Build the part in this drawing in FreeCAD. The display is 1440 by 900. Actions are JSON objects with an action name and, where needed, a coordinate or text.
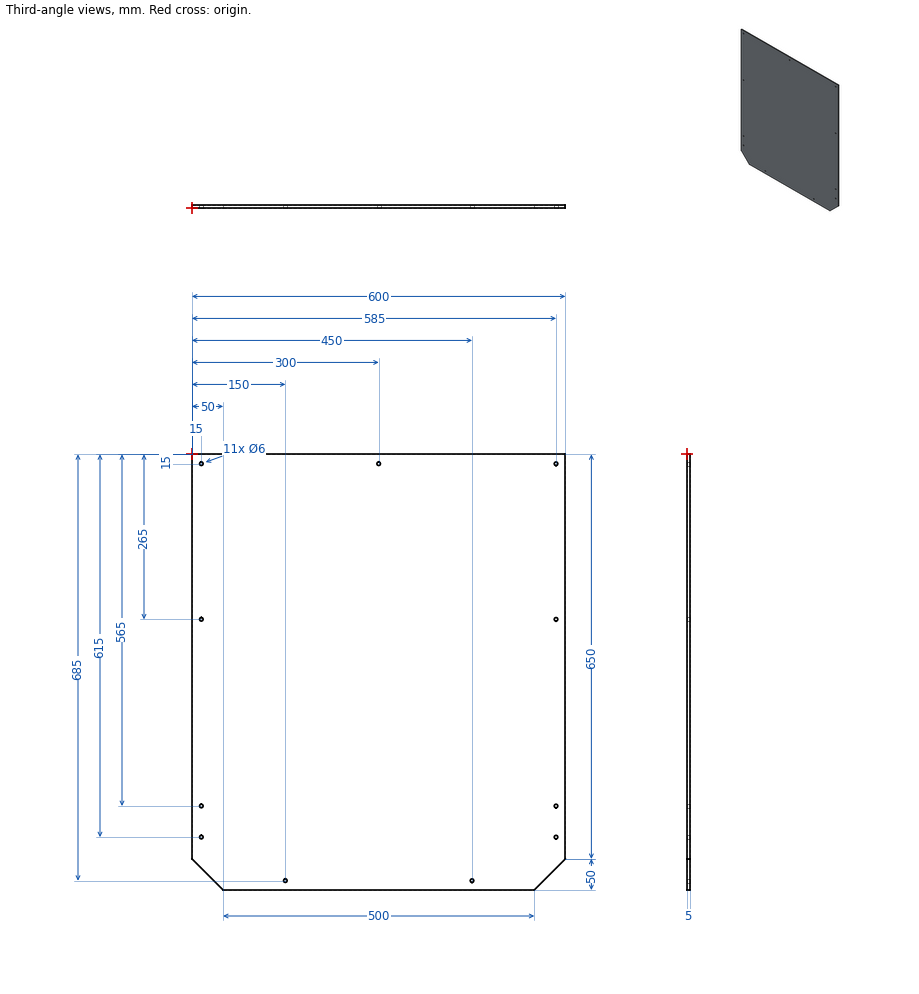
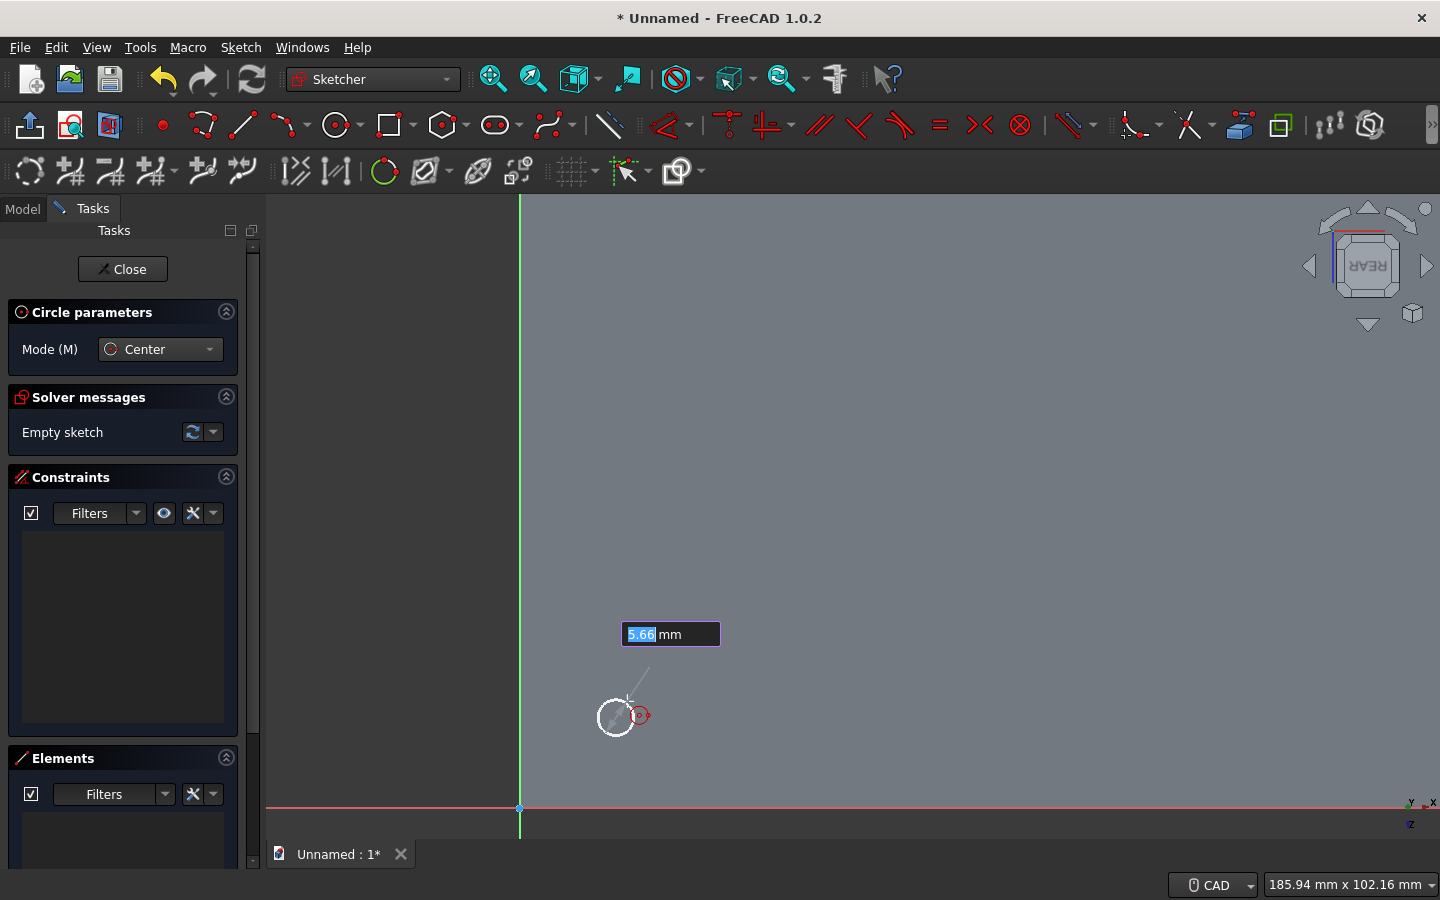
{"action": "left_click", "coordinate": [628, 700]}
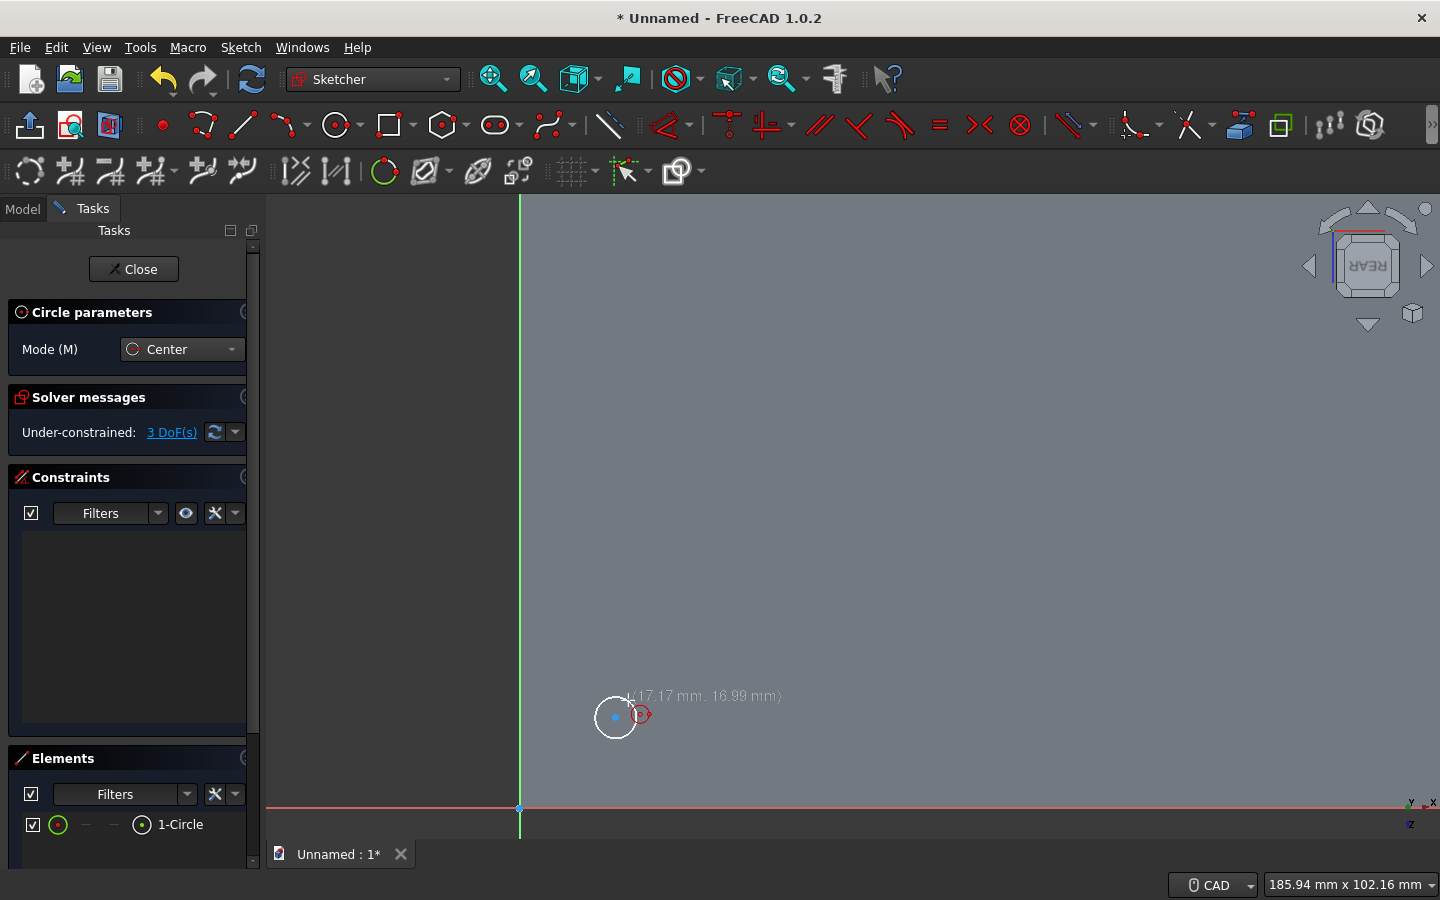
{"action": "scroll", "coordinate": [626, 704], "scroll_direction": "down", "scroll_amount": 12}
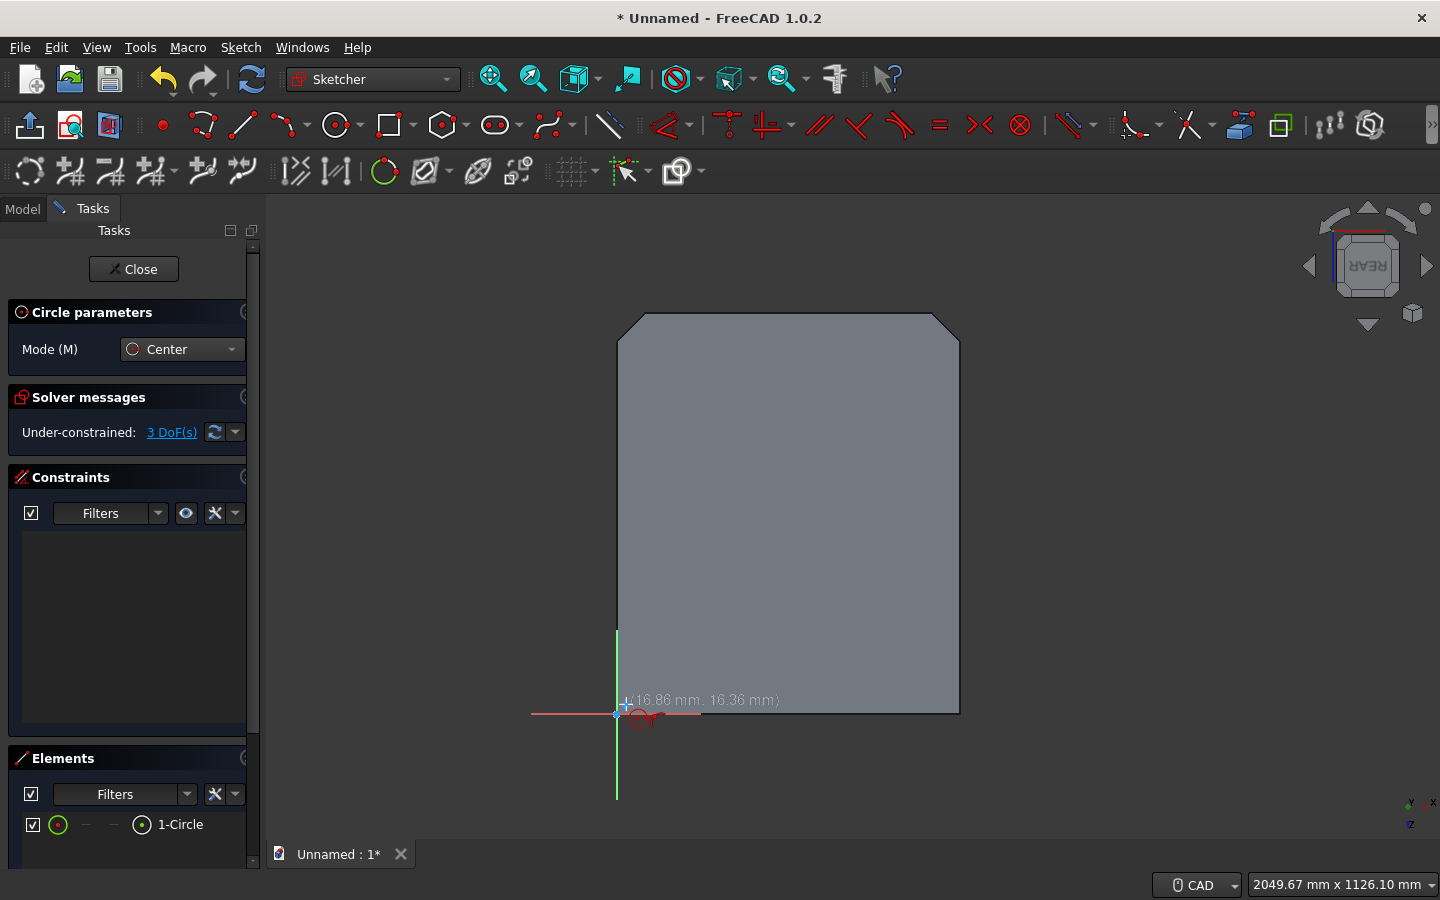
{"action": "scroll", "coordinate": [625, 562], "scroll_direction": "up", "scroll_amount": 13}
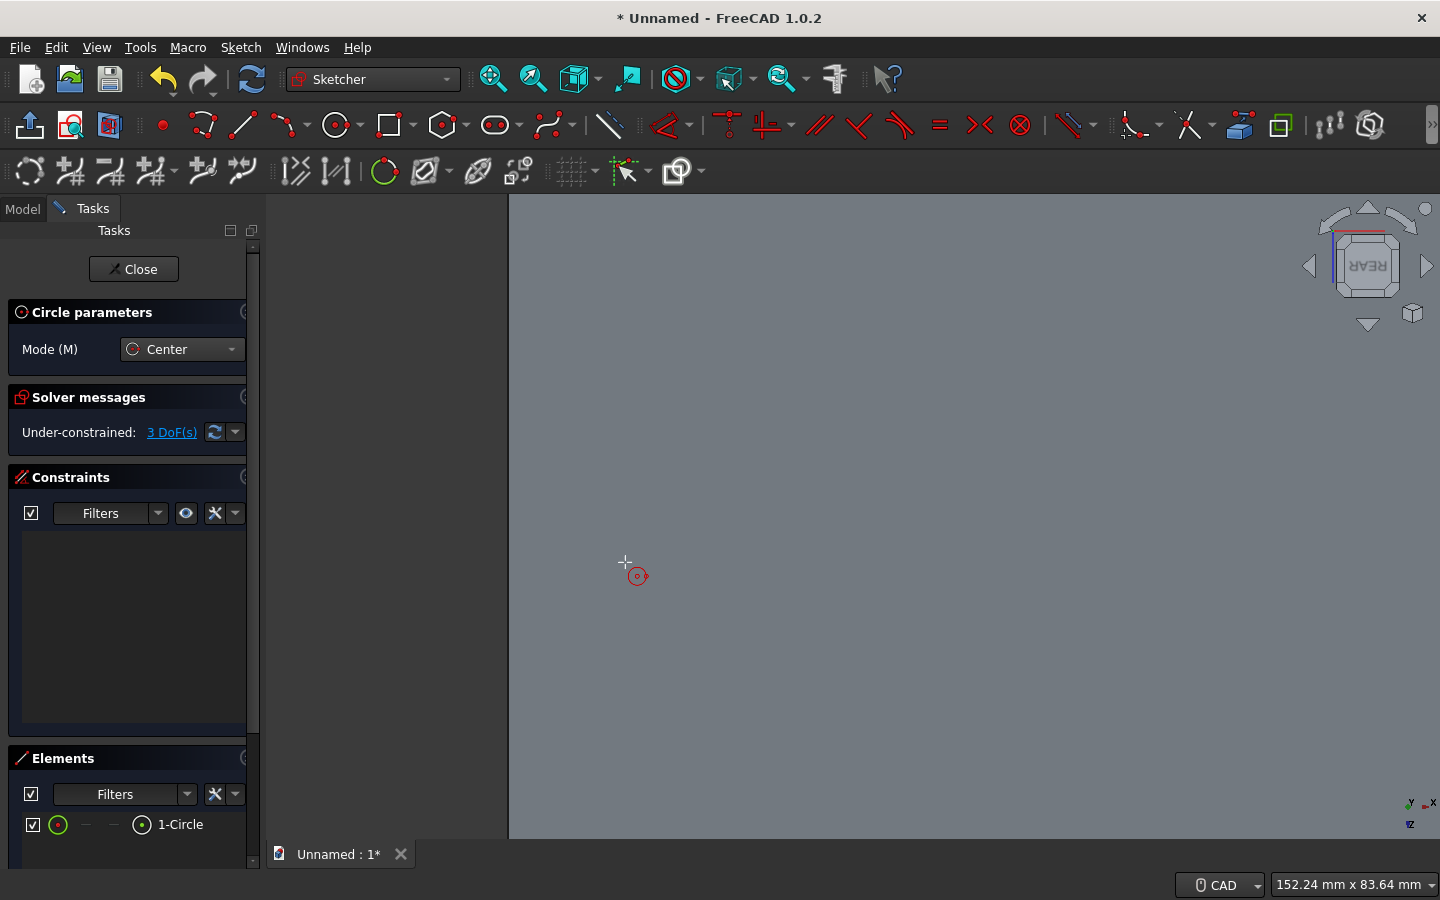
{"action": "scroll", "coordinate": [625, 562], "scroll_direction": "down", "scroll_amount": 13}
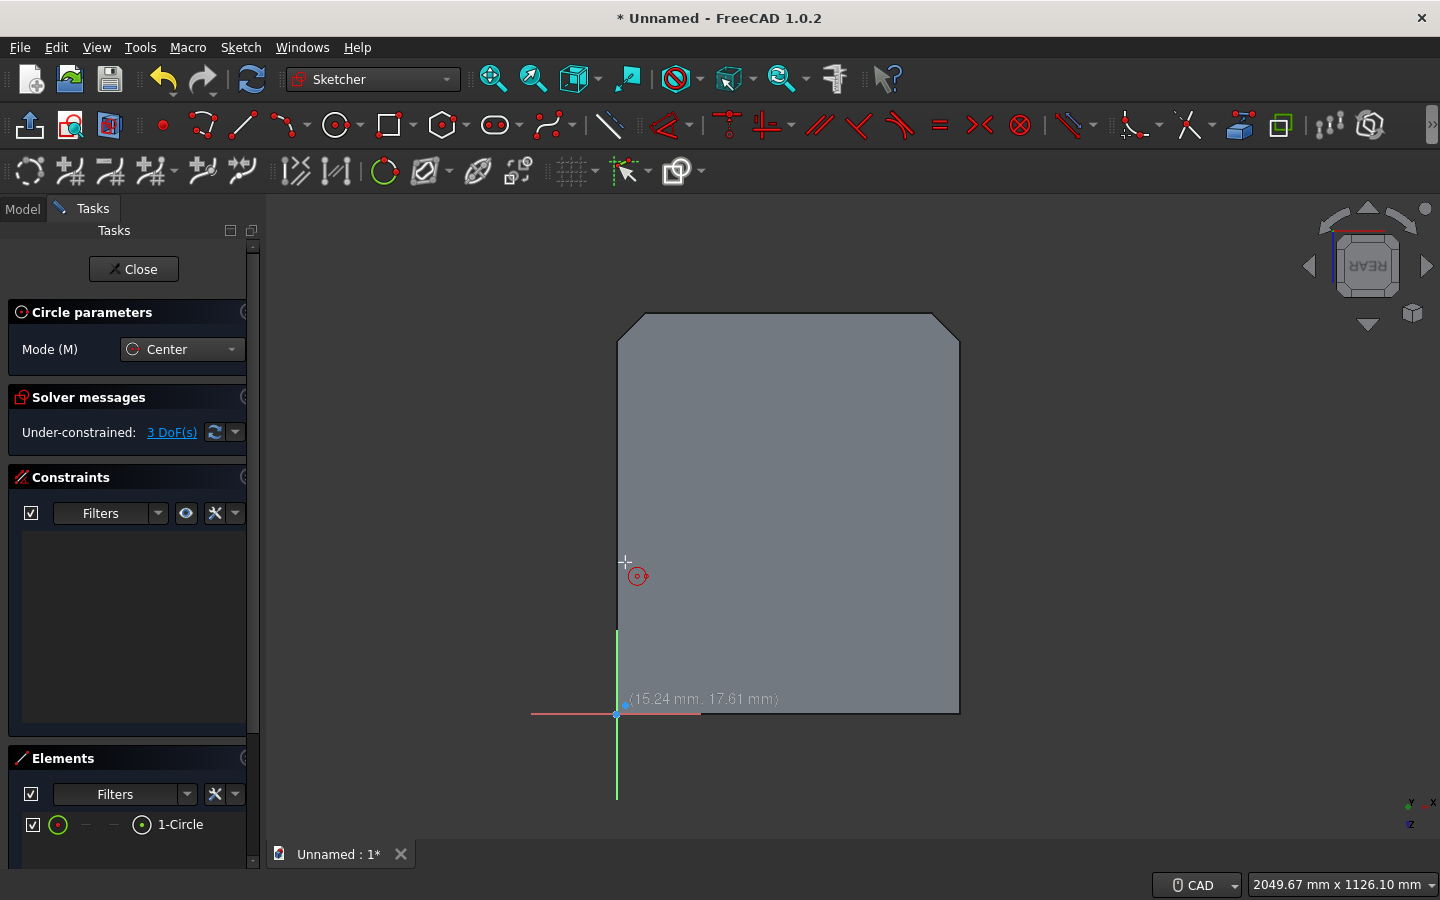
{"action": "scroll", "coordinate": [625, 562], "scroll_direction": "up", "scroll_amount": 4}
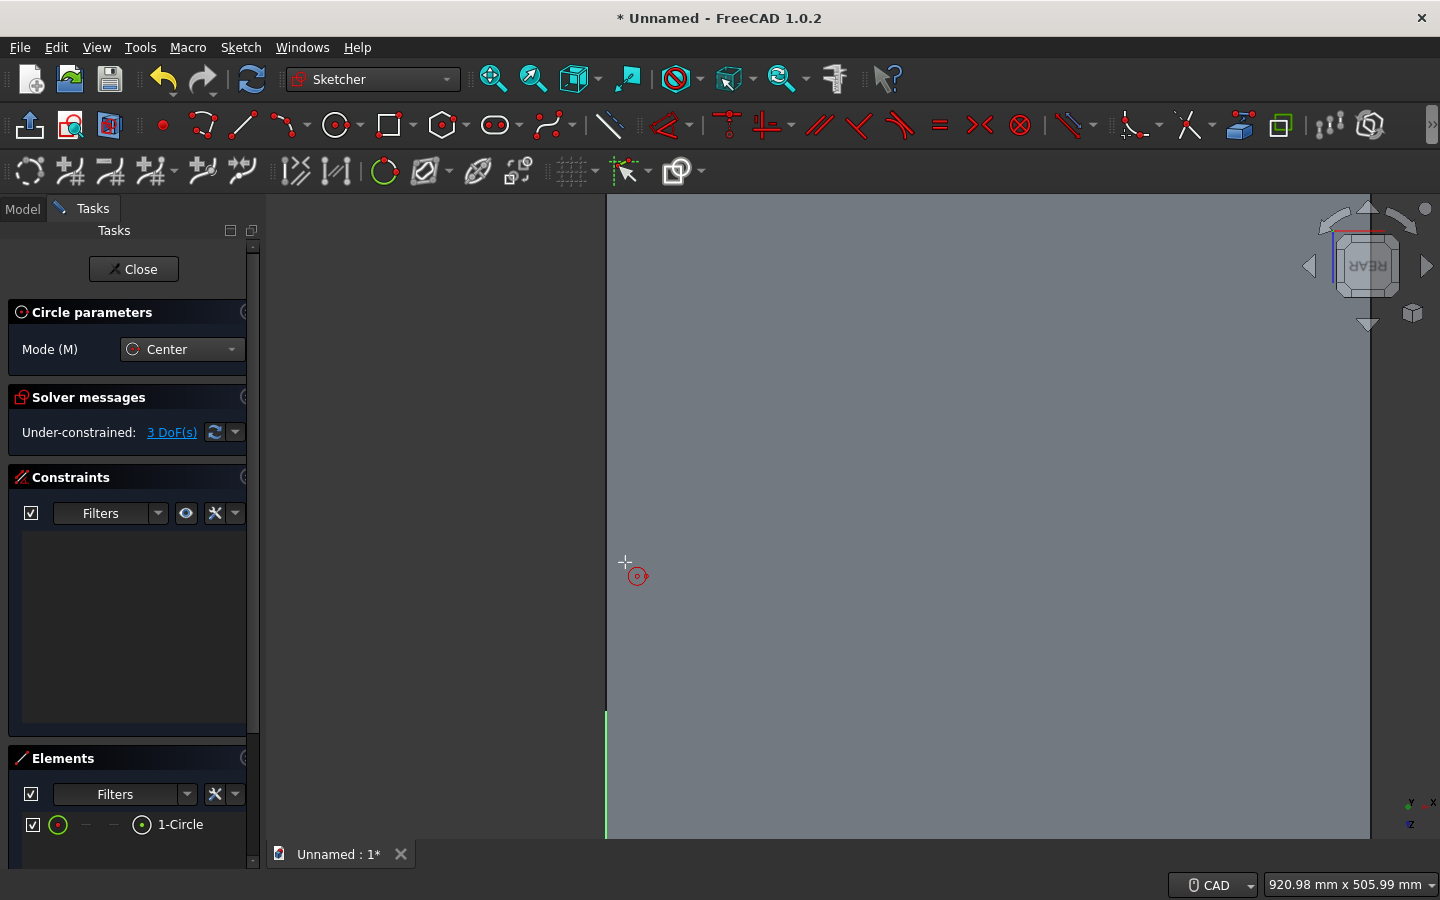
{"action": "left_click", "coordinate": [625, 562]}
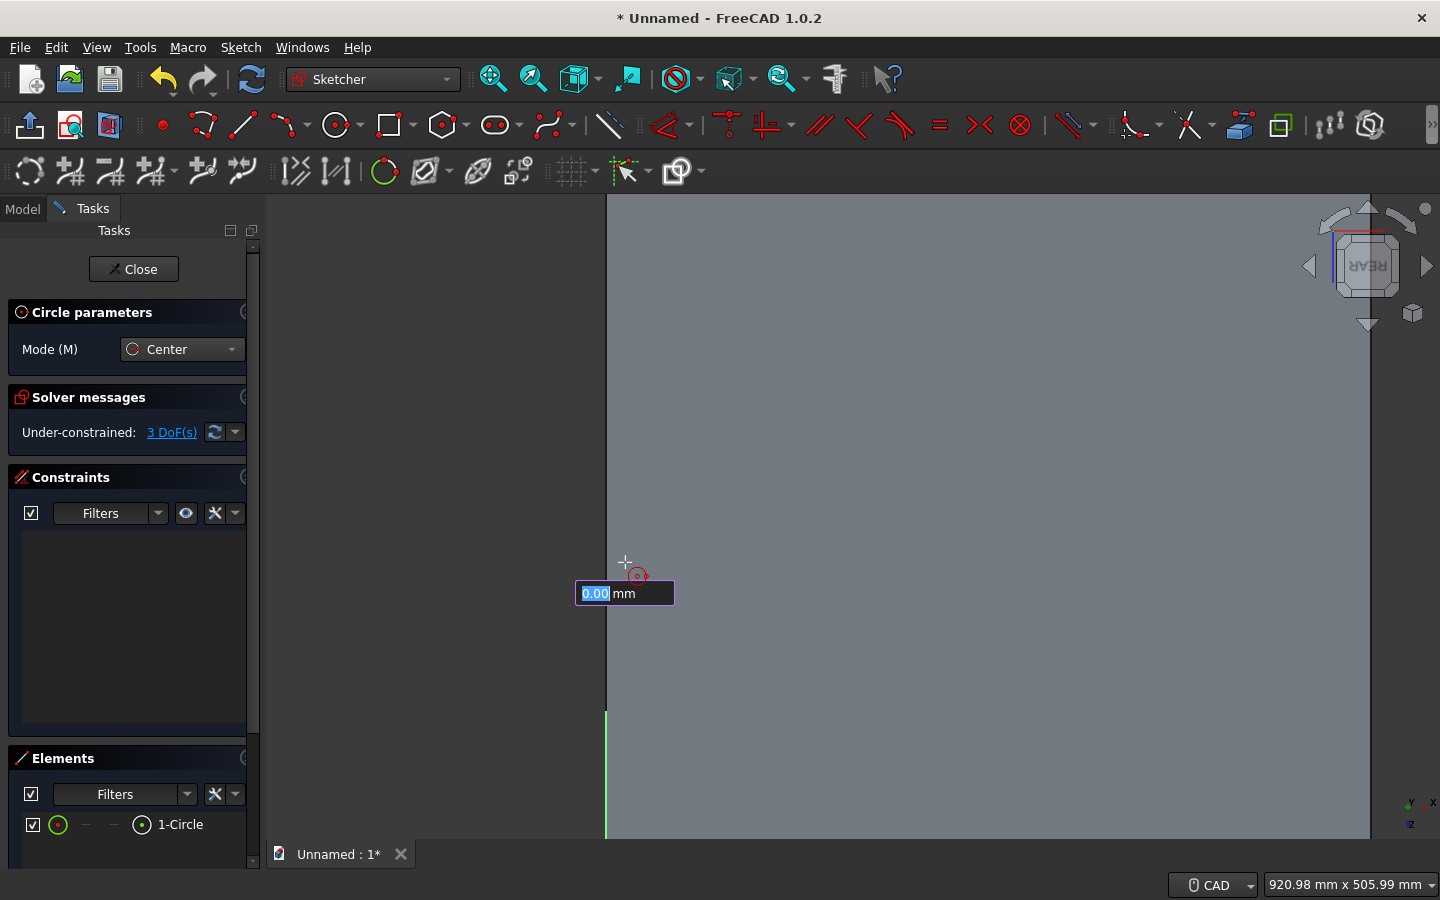
{"action": "scroll", "coordinate": [628, 559], "scroll_direction": "up", "scroll_amount": 8}